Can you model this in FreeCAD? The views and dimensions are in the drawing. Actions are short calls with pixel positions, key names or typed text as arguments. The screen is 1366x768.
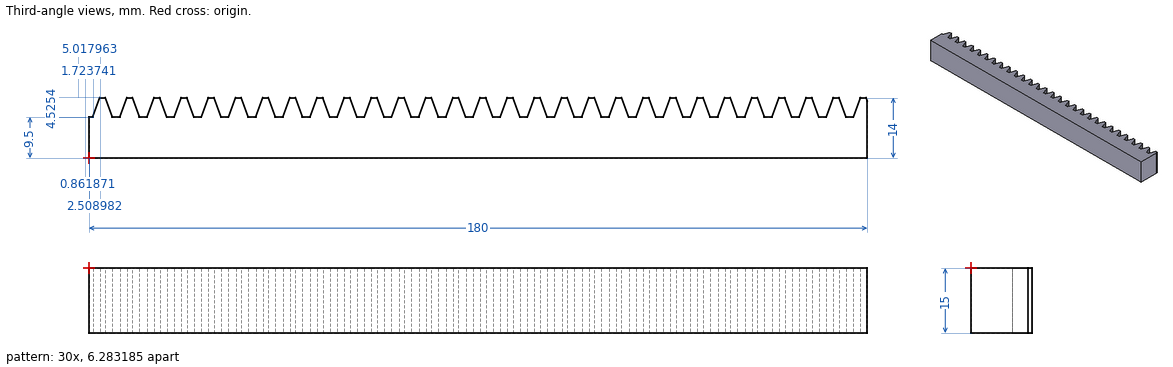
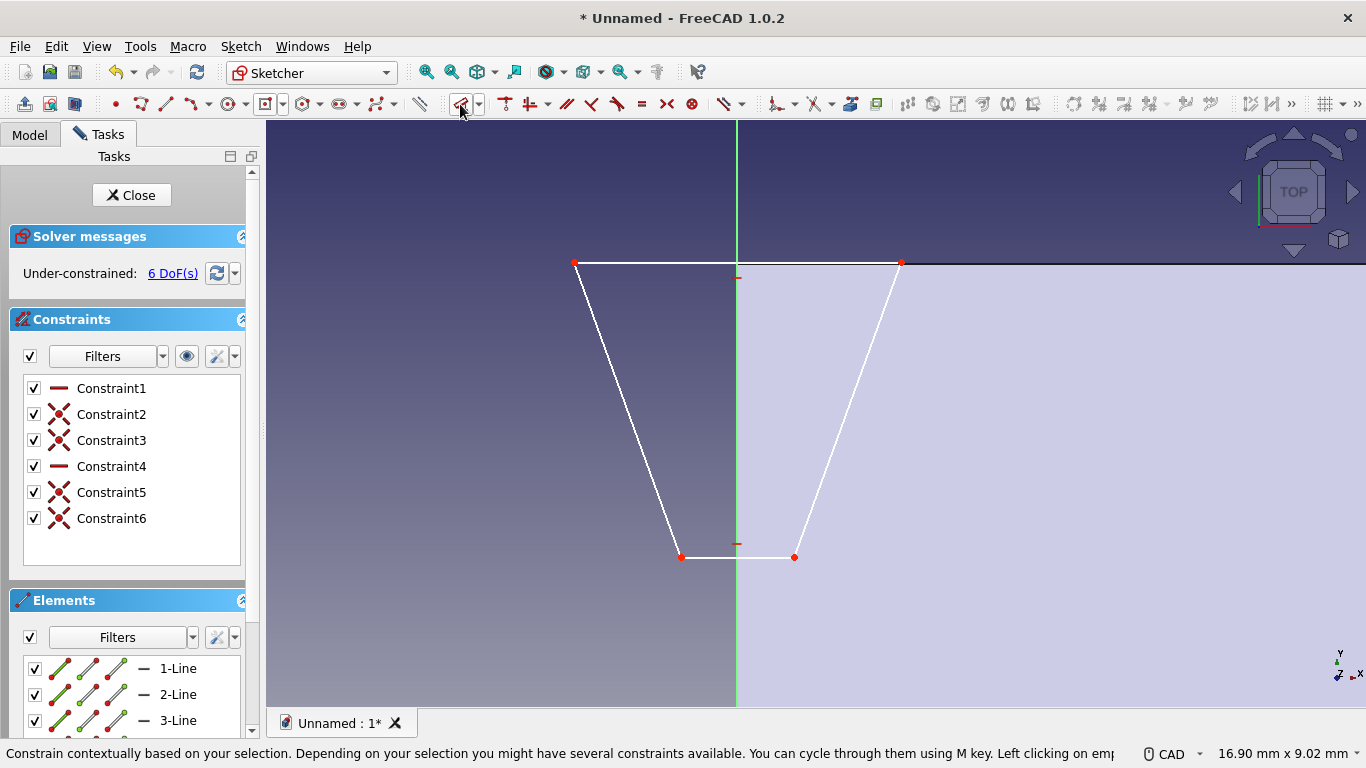
click(681, 558)
click(647, 618)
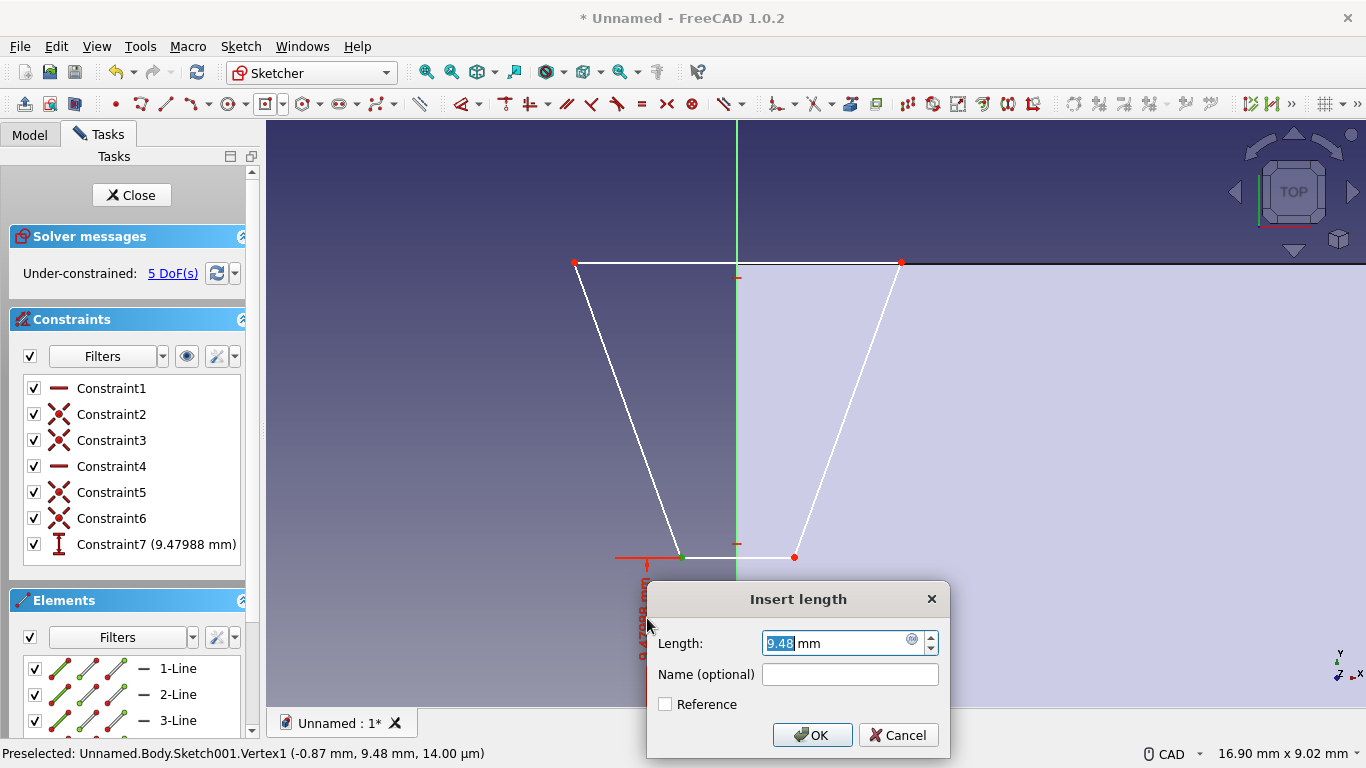
text(9.5)
key(Return)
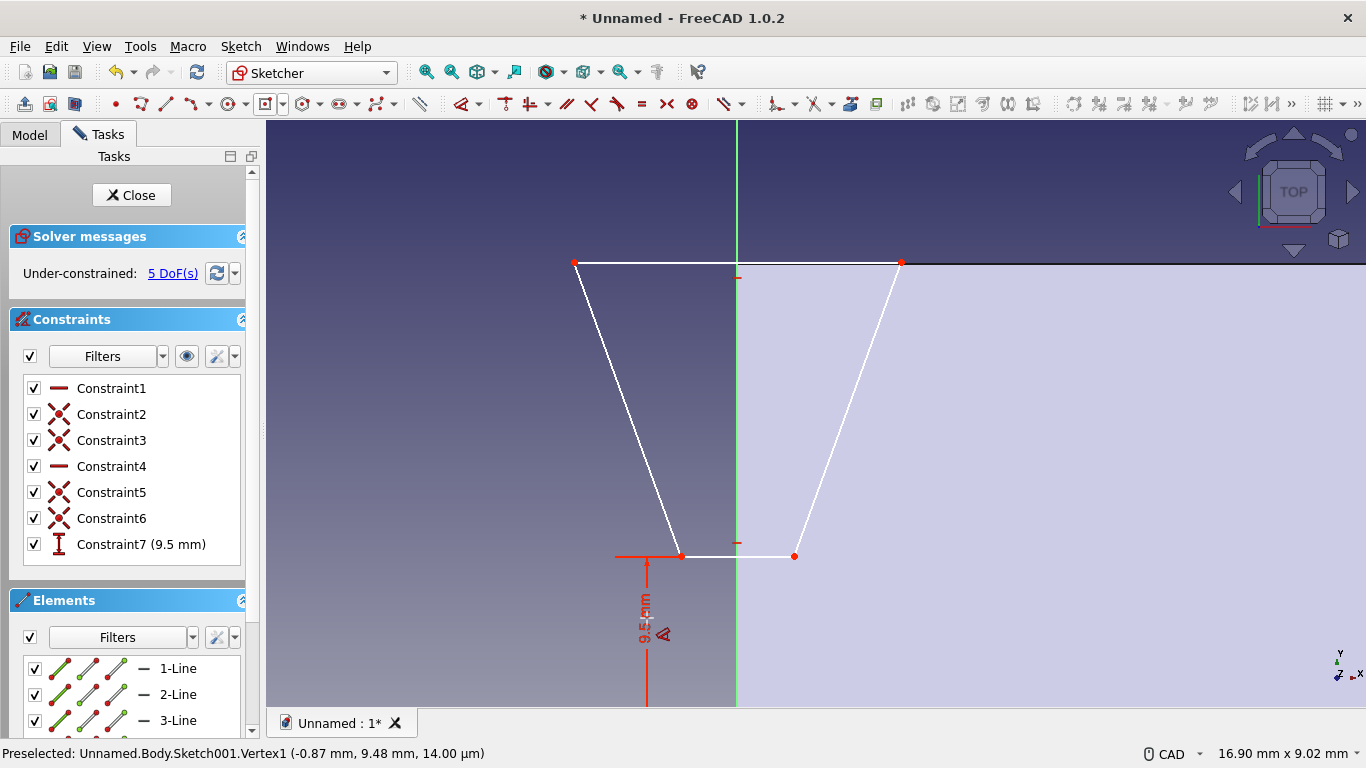
click(826, 469)
click(935, 410)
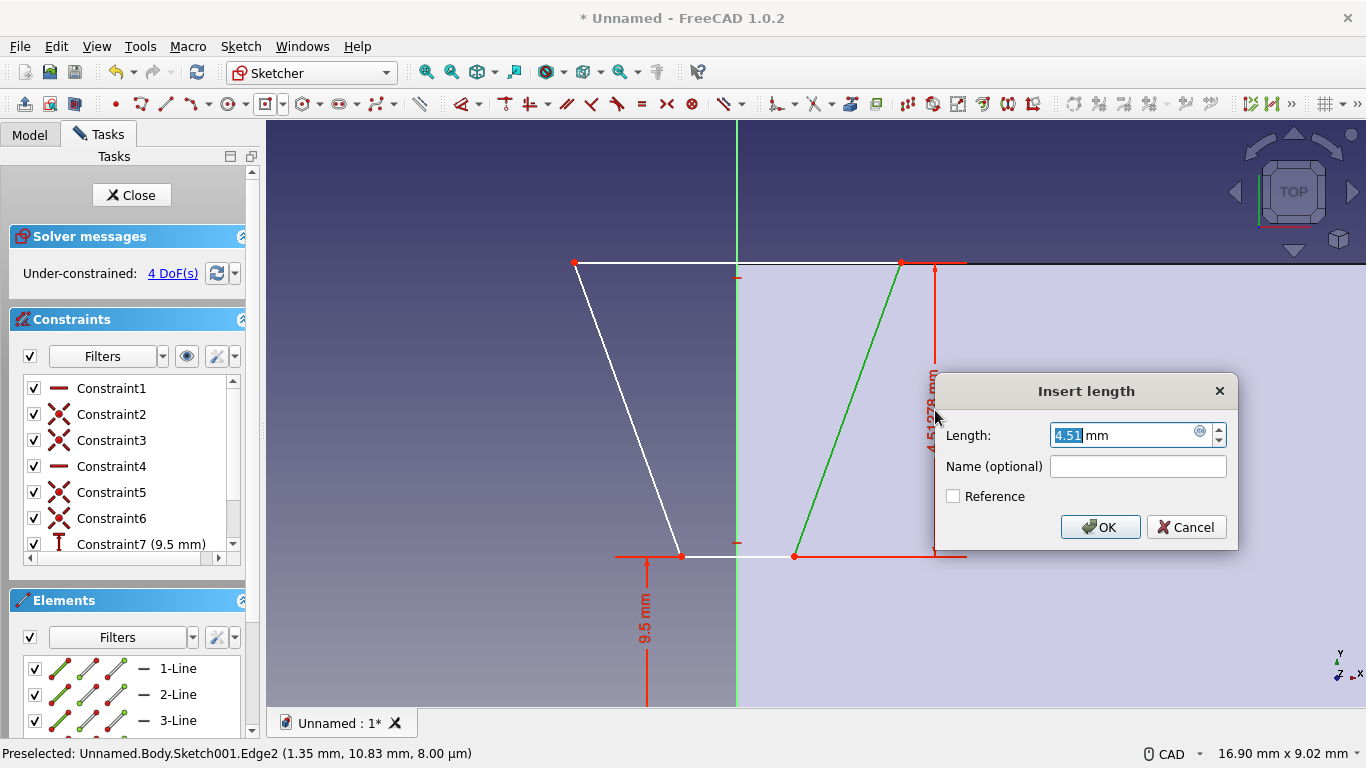
text(4.5254)
key(Return)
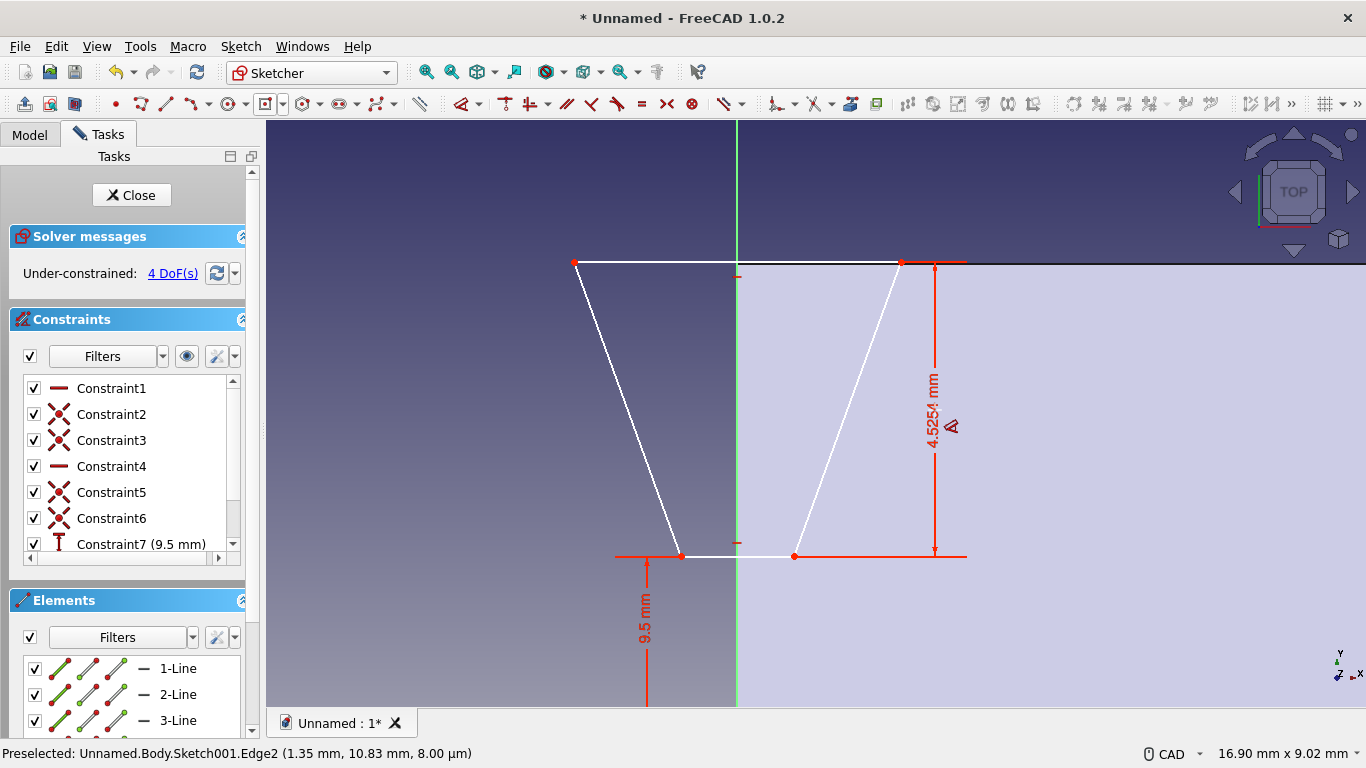
click(715, 557)
click(712, 591)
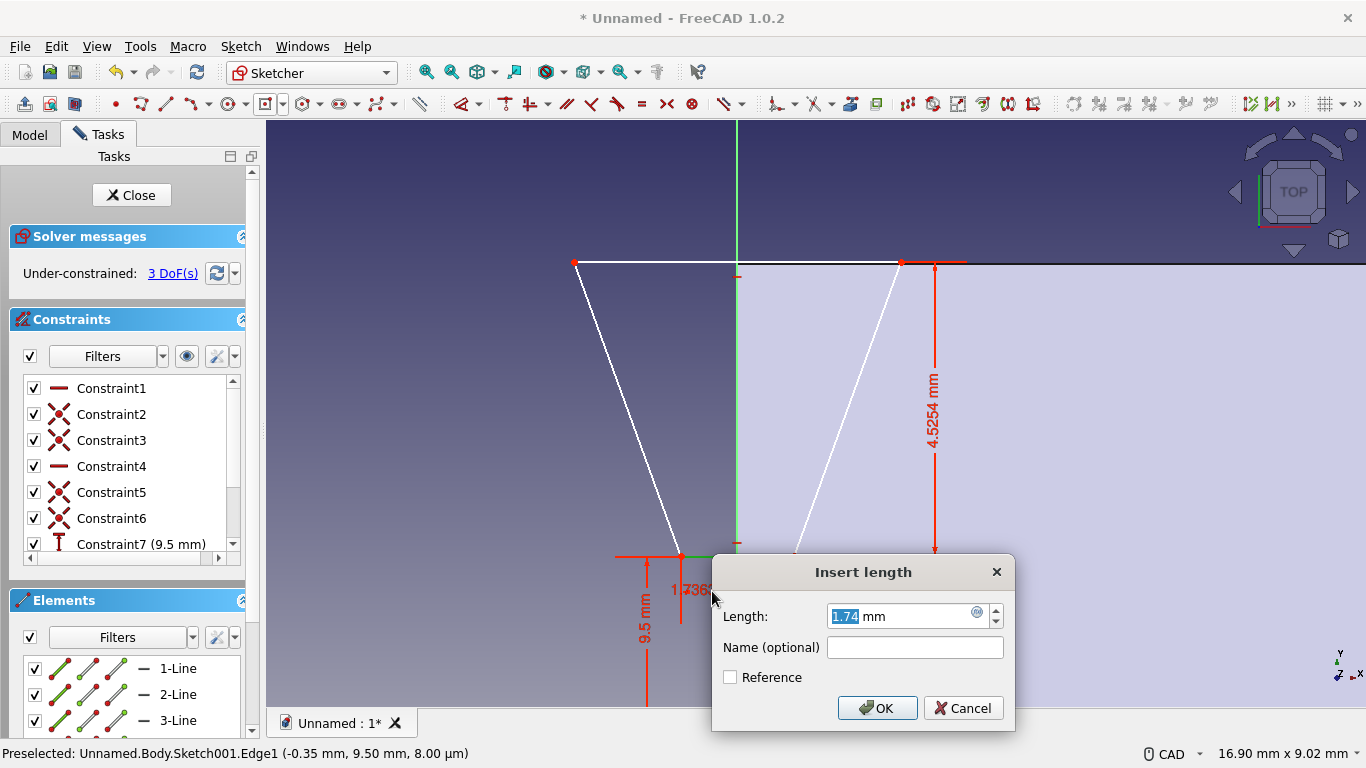
text(1.723741)
key(Return)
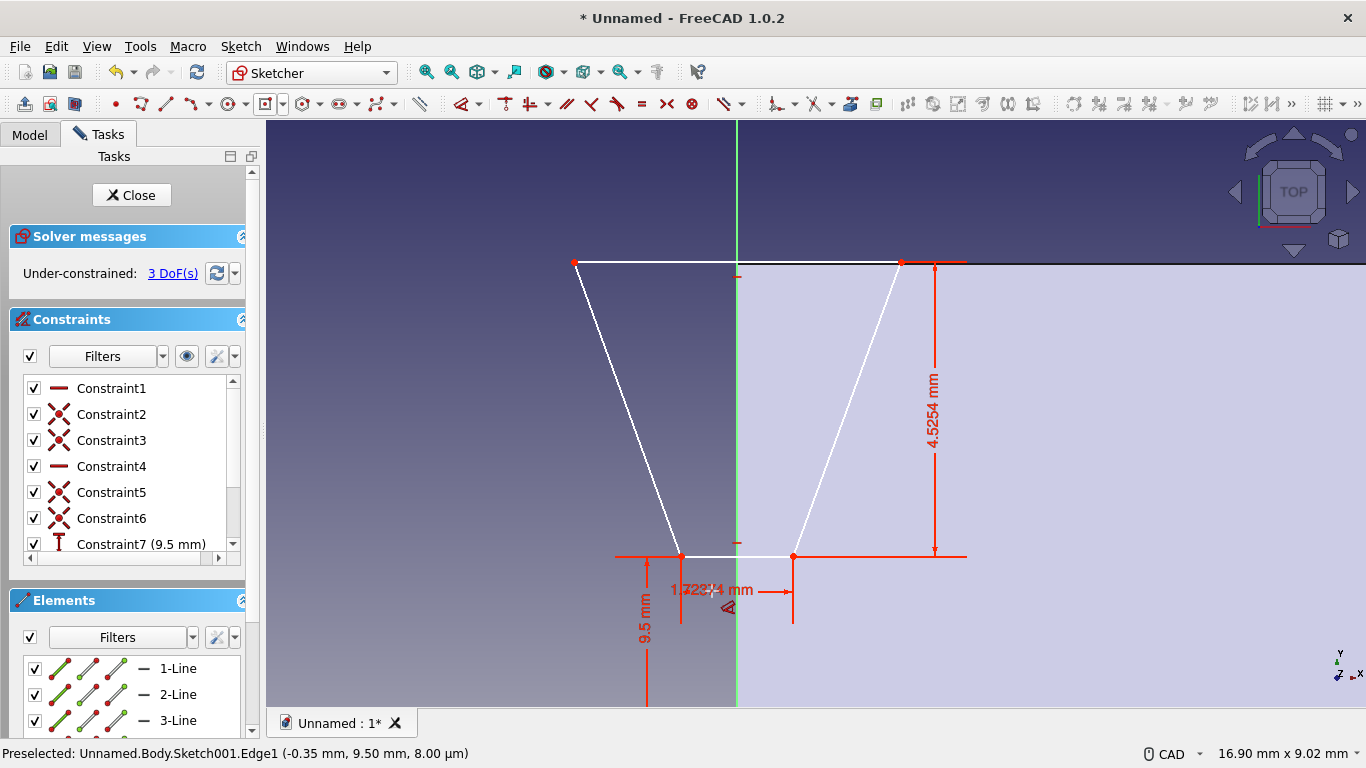
click(803, 262)
click(662, 228)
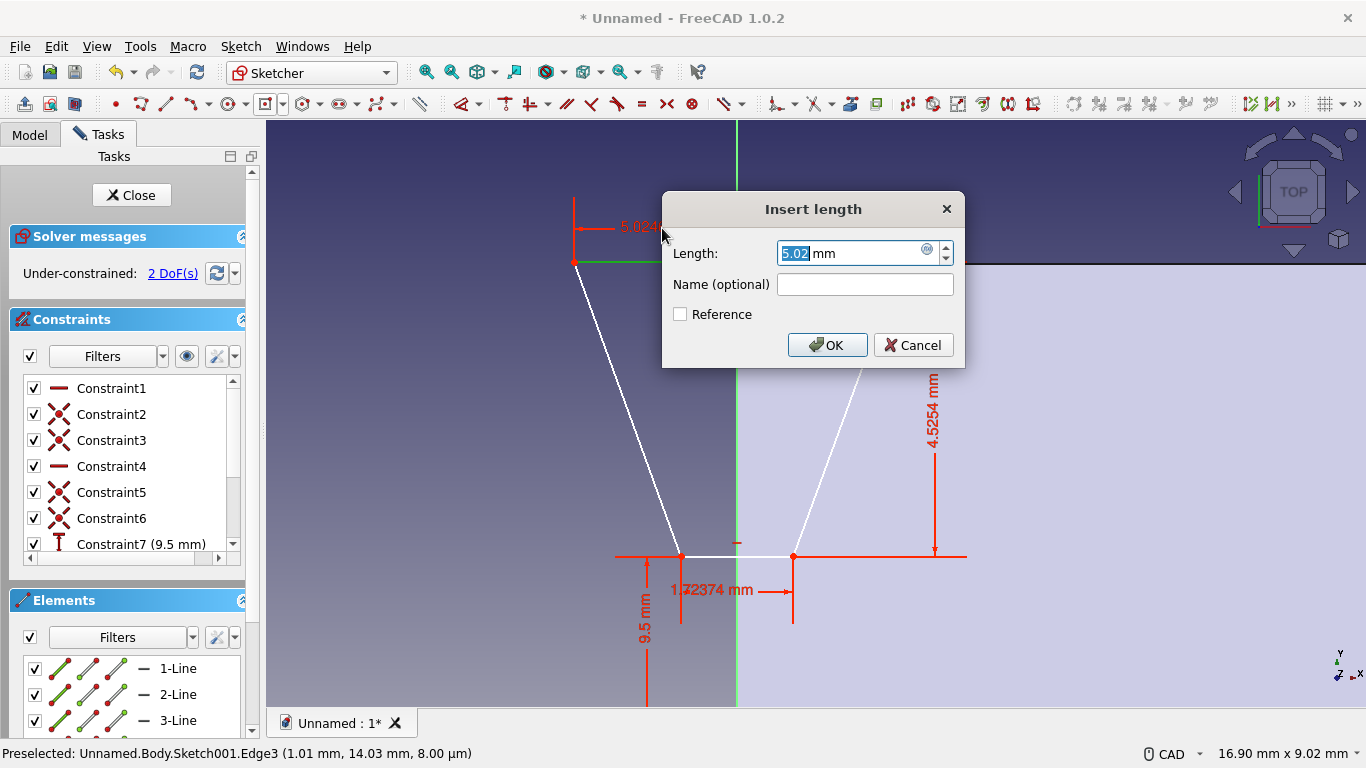
text(5.017963)
key(Return)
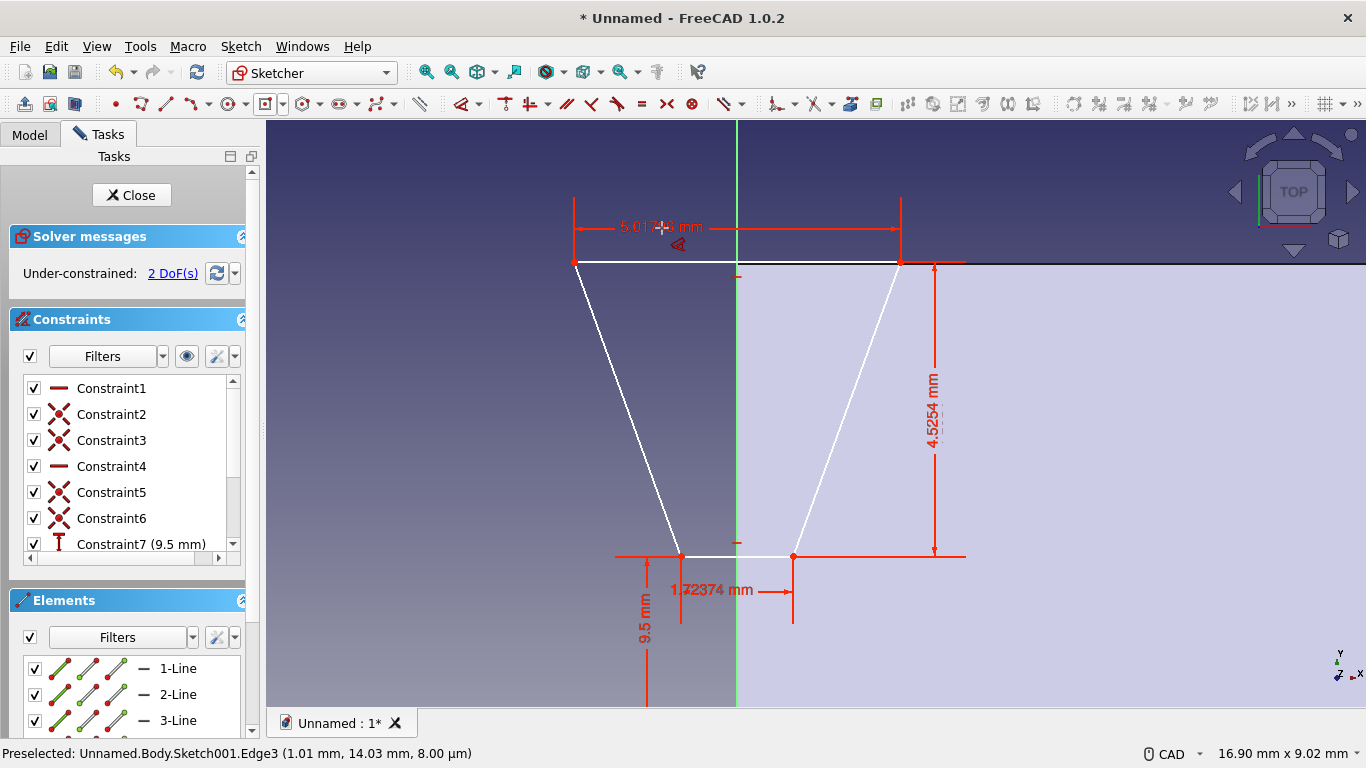
click(681, 557)
click(709, 523)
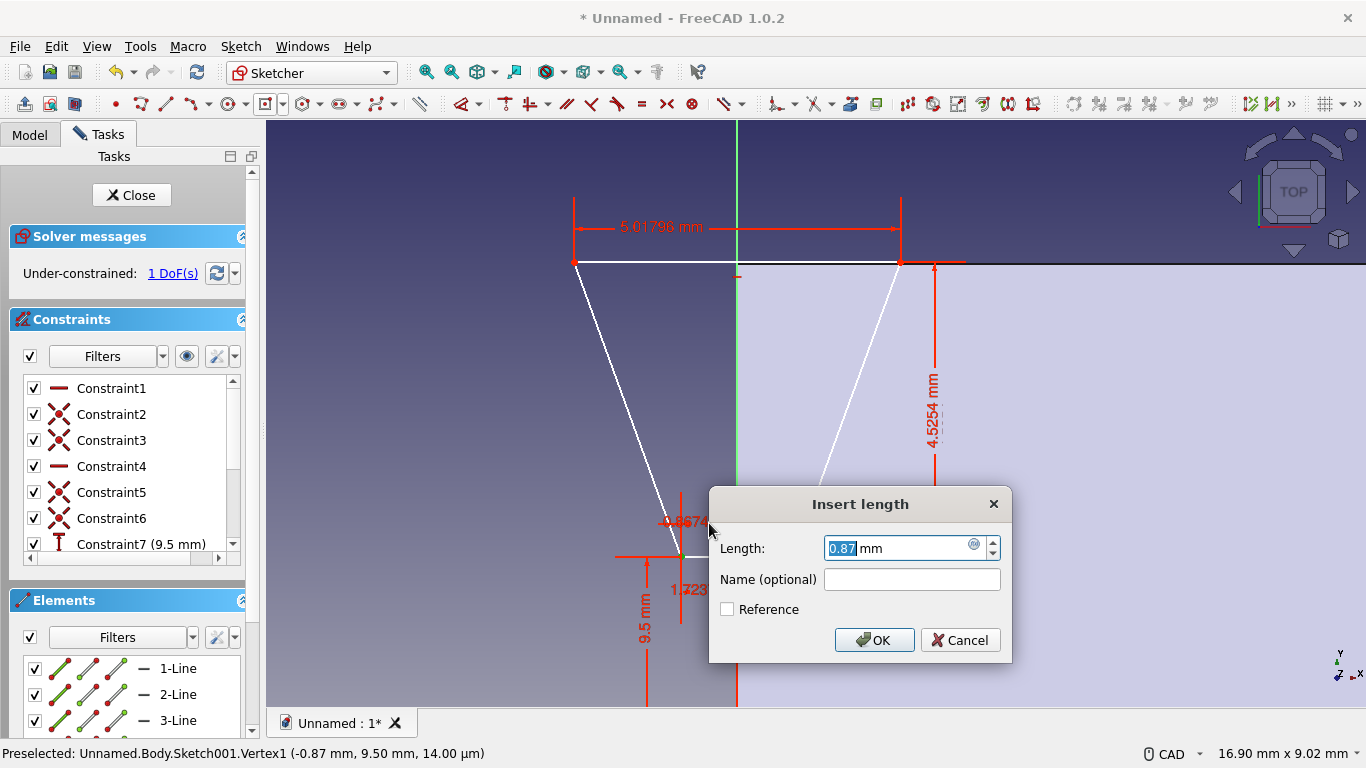
text(0.861871)
key(Return)